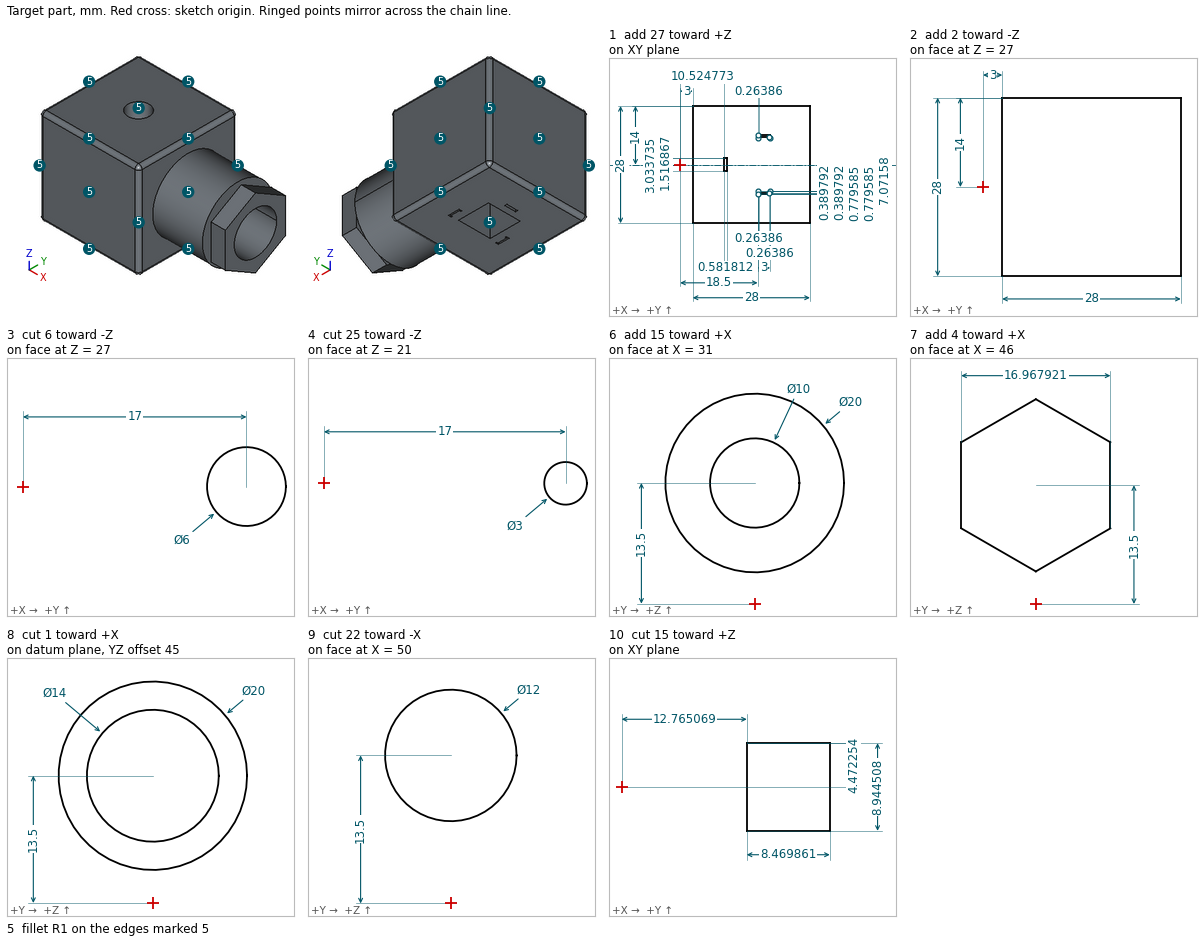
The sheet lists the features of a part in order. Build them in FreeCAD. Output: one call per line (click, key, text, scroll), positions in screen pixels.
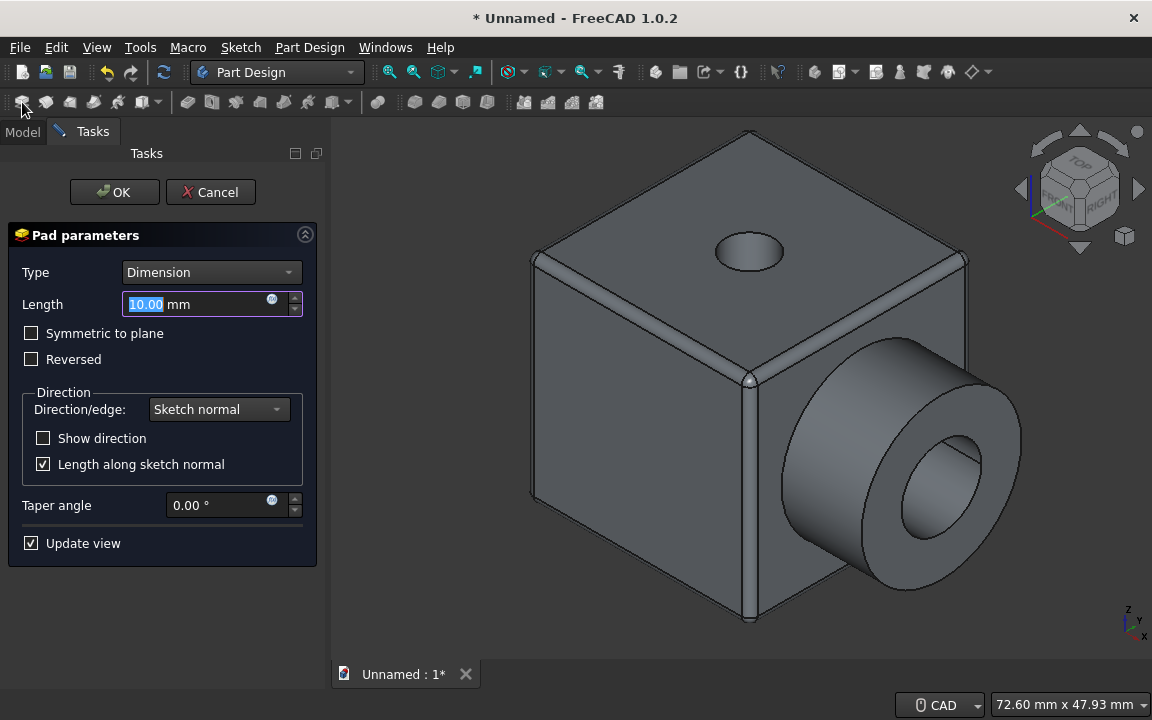
text(15)
key(Tab)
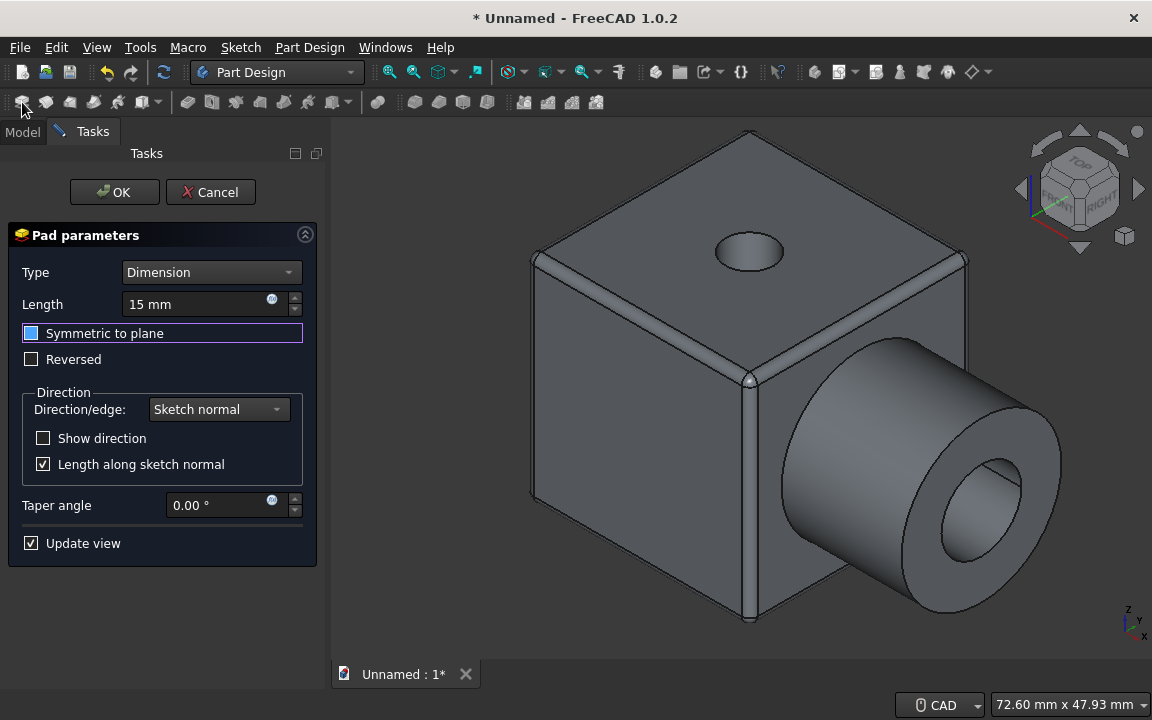
click(115, 192)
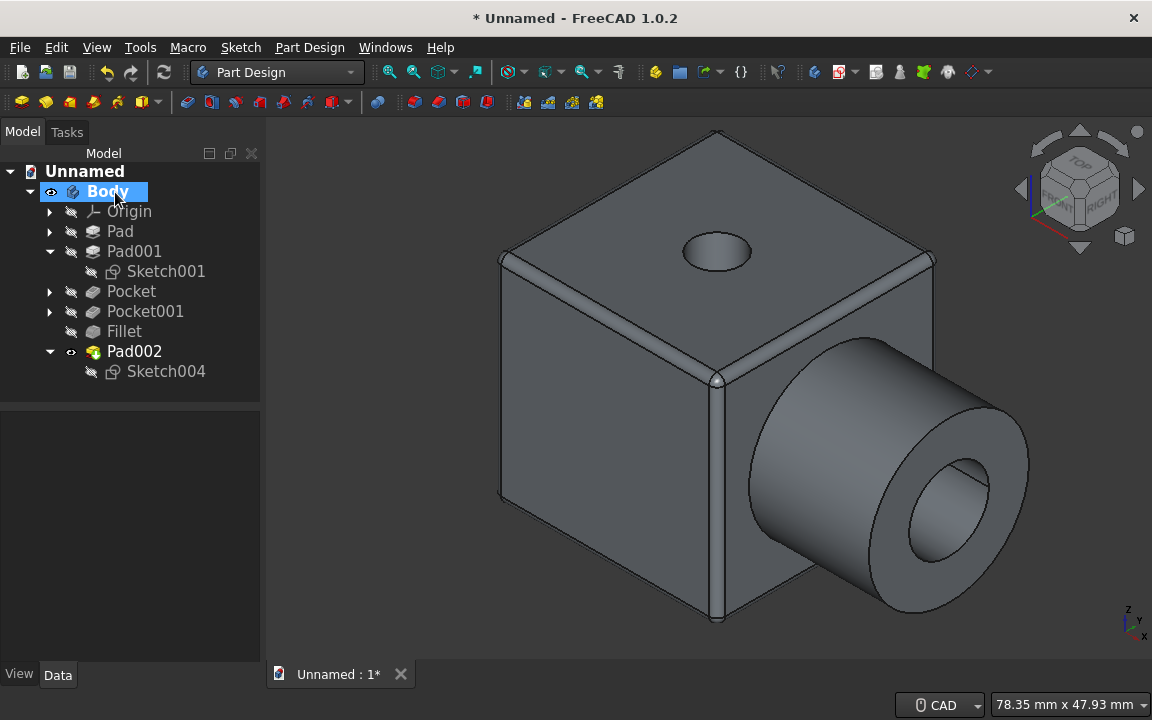
click(390, 72)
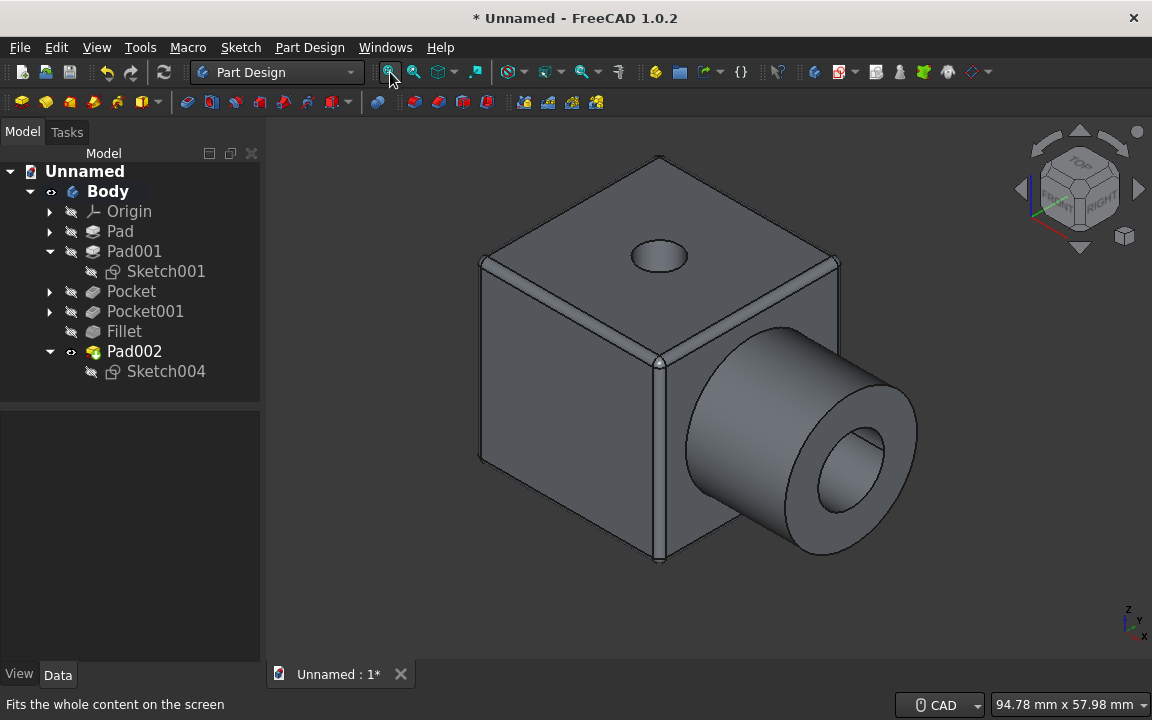
click(813, 534)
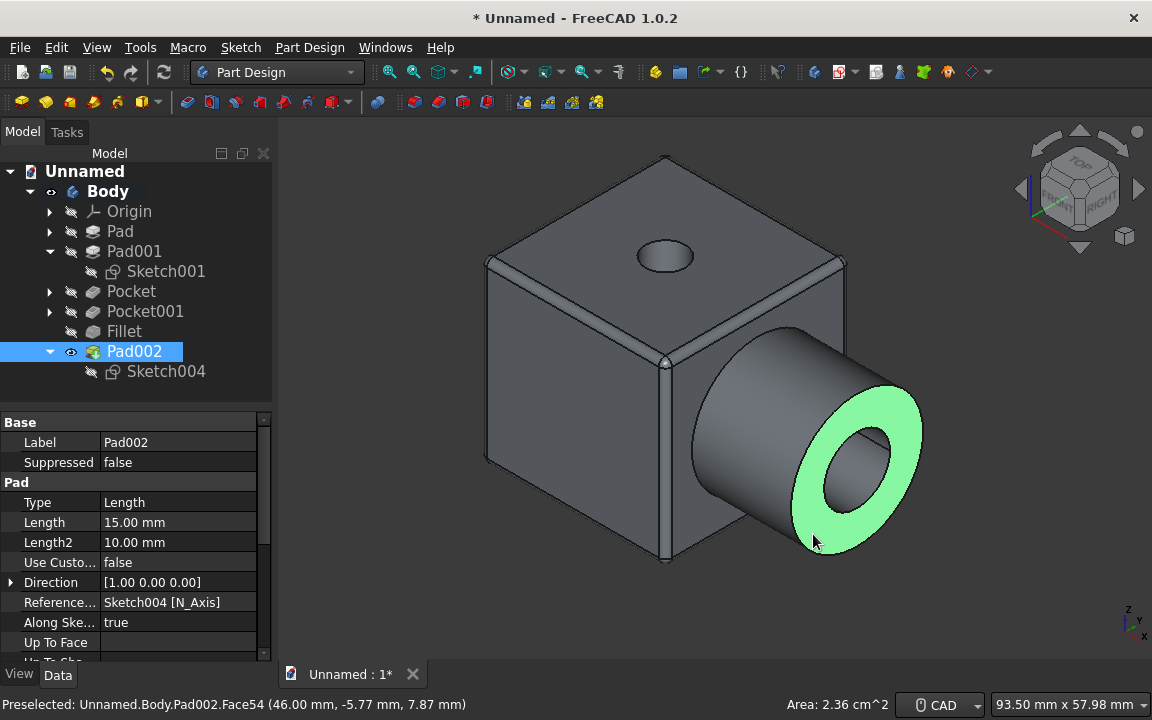
click(840, 72)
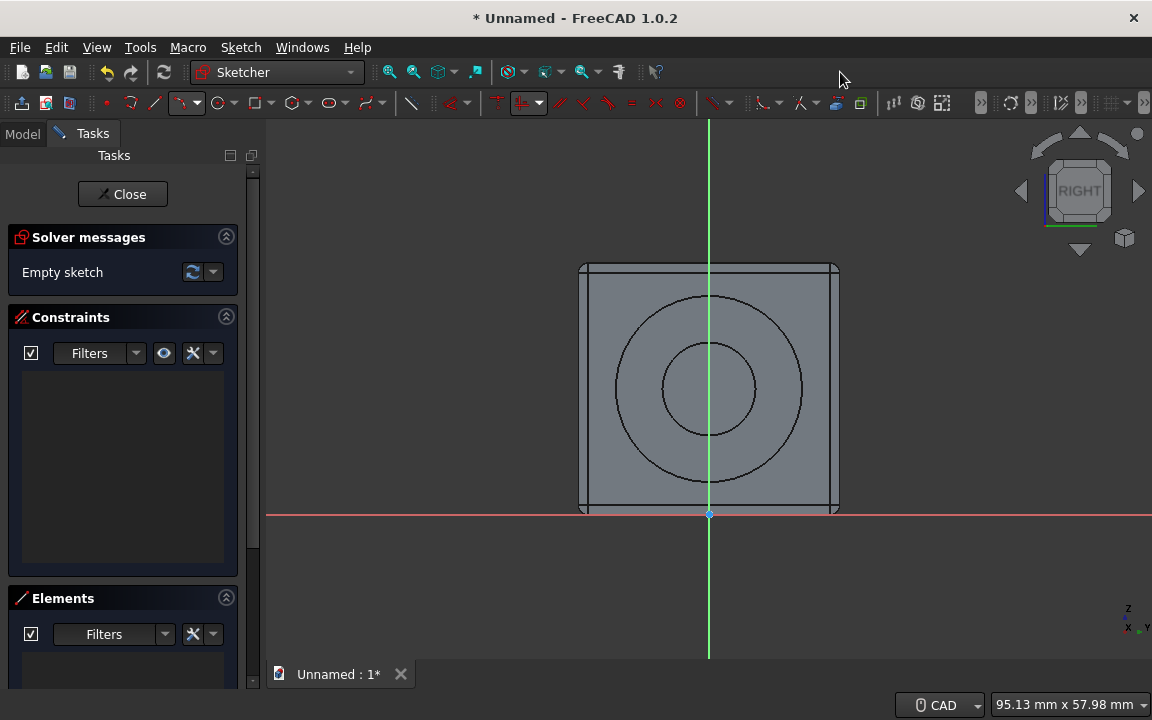
scroll(848, 441, up, 2)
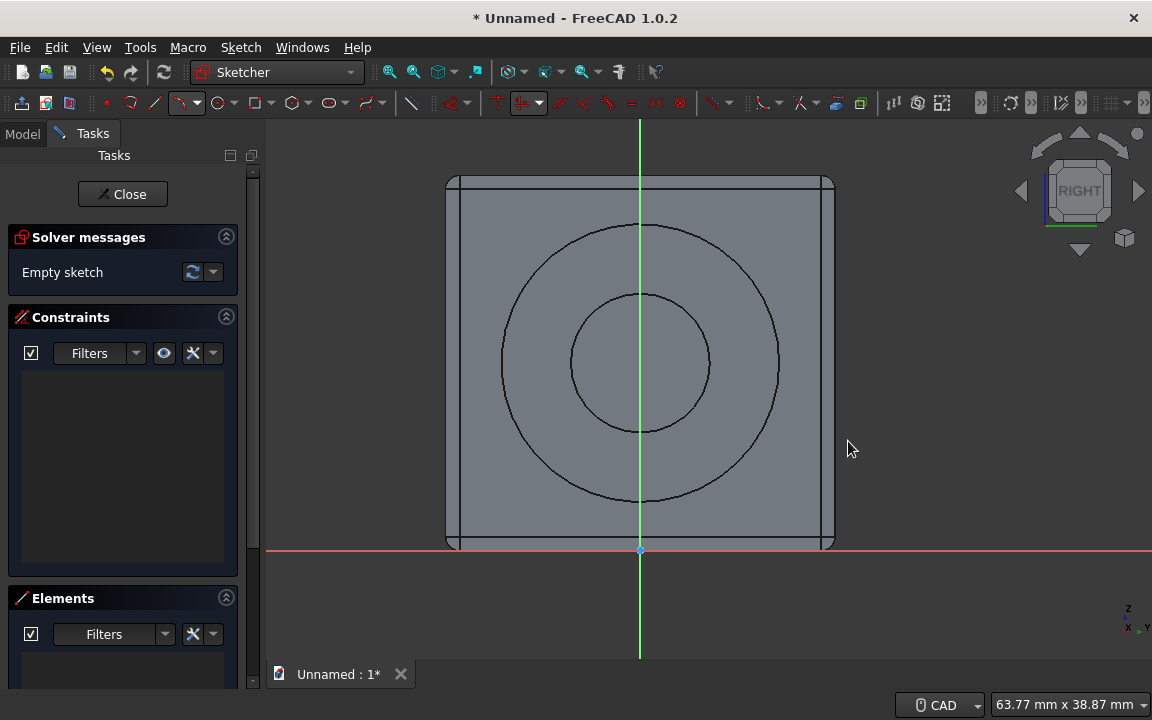
click(292, 104)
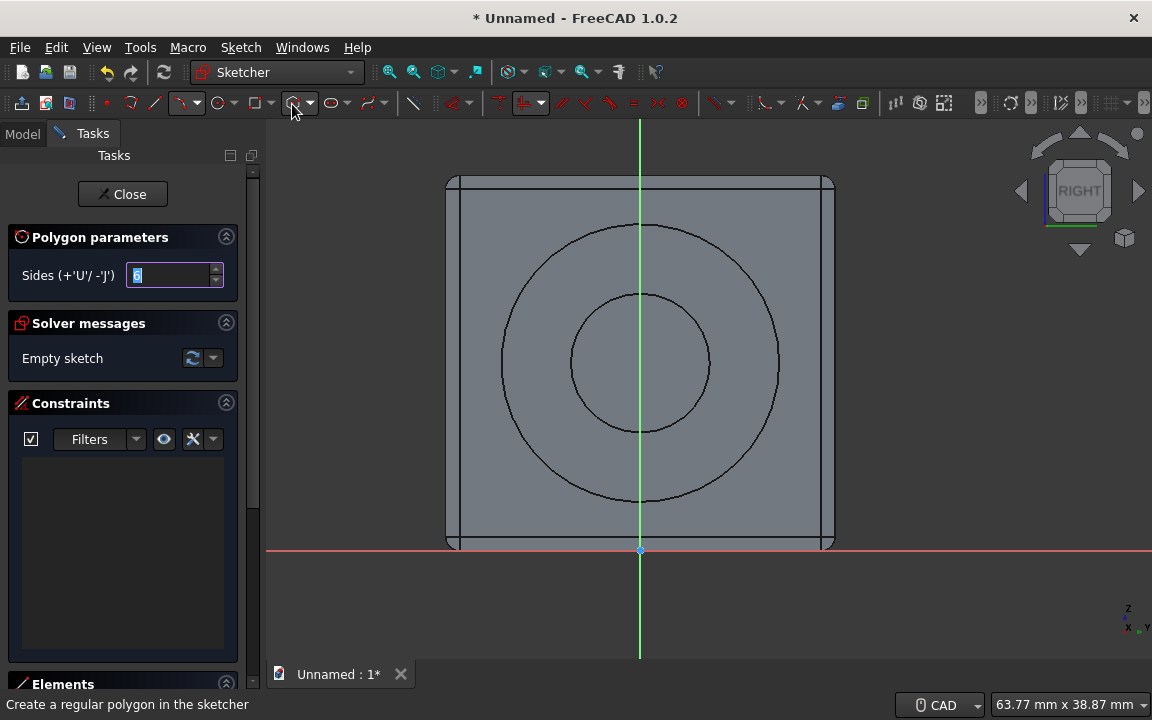
click(640, 363)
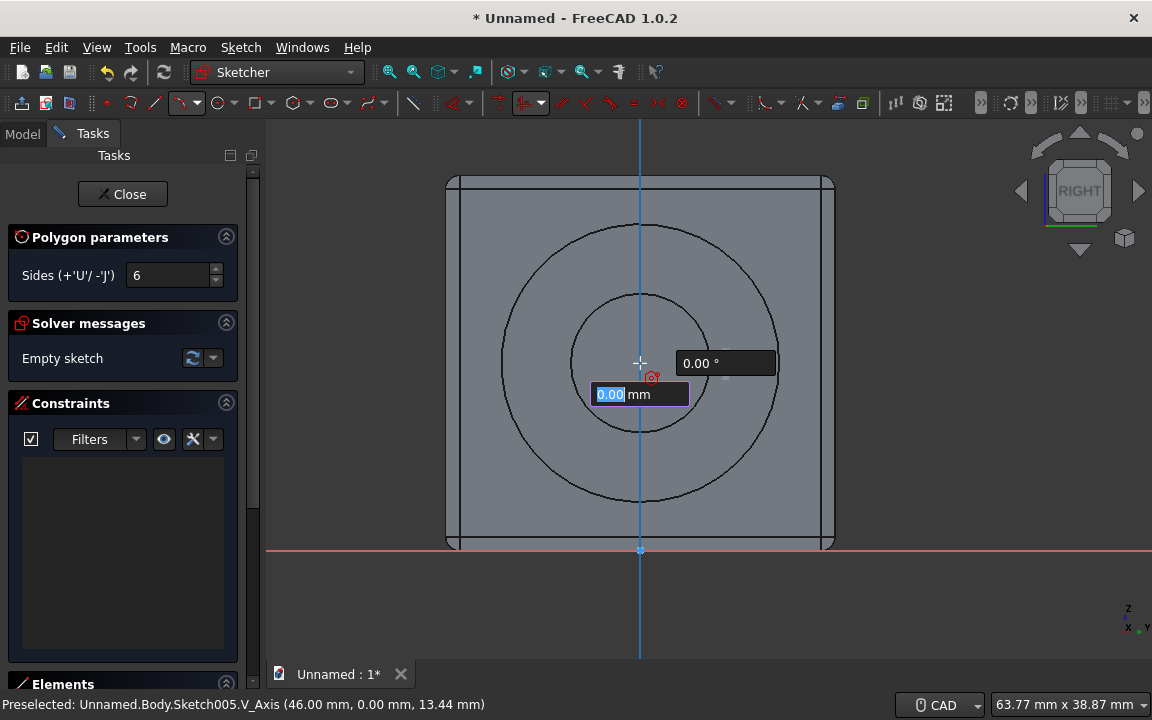
click(640, 227)
right_click(640, 227)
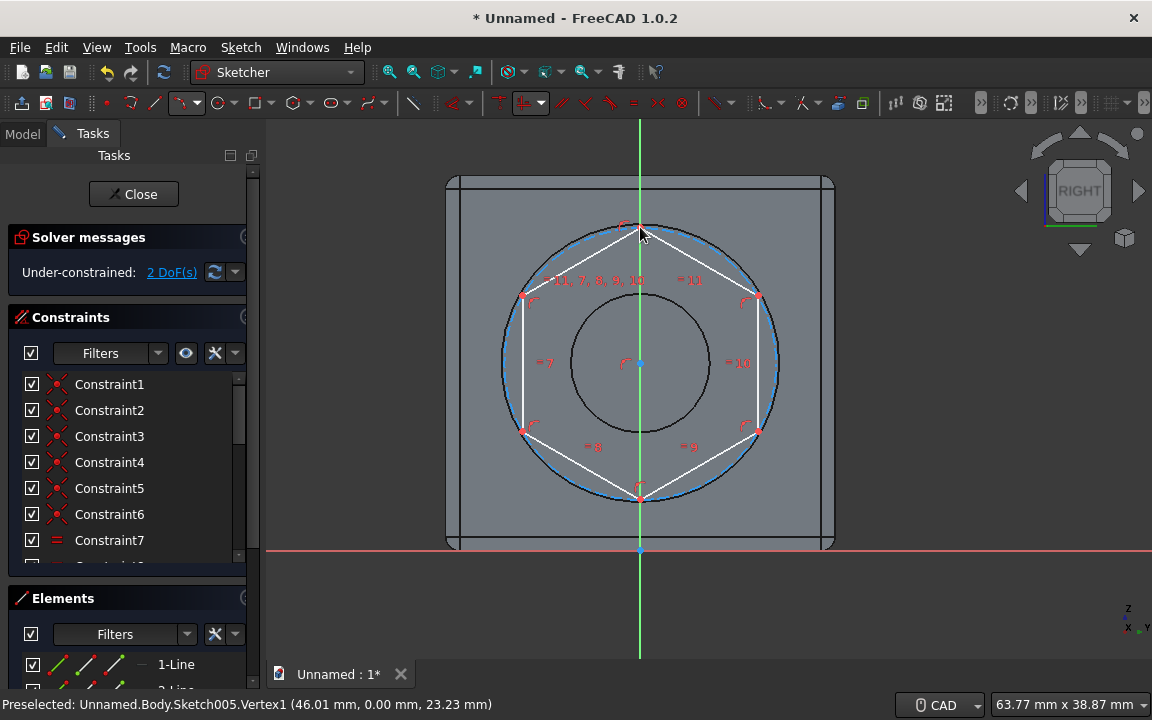
click(452, 104)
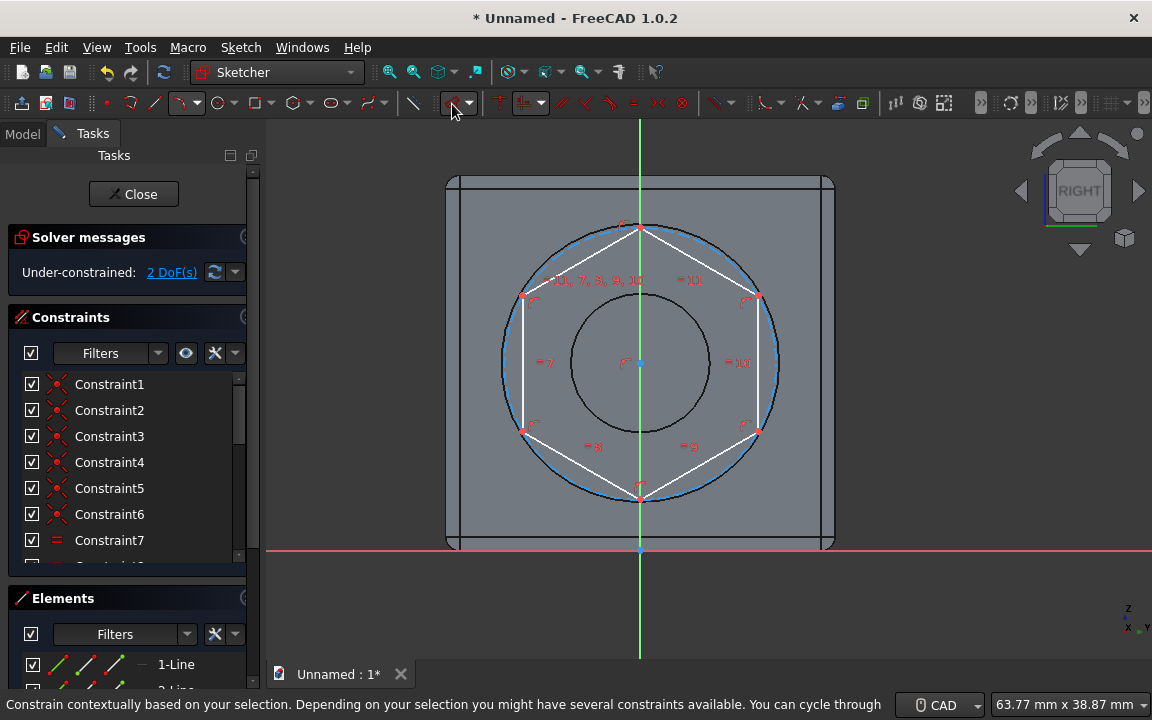
click(640, 364)
click(674, 457)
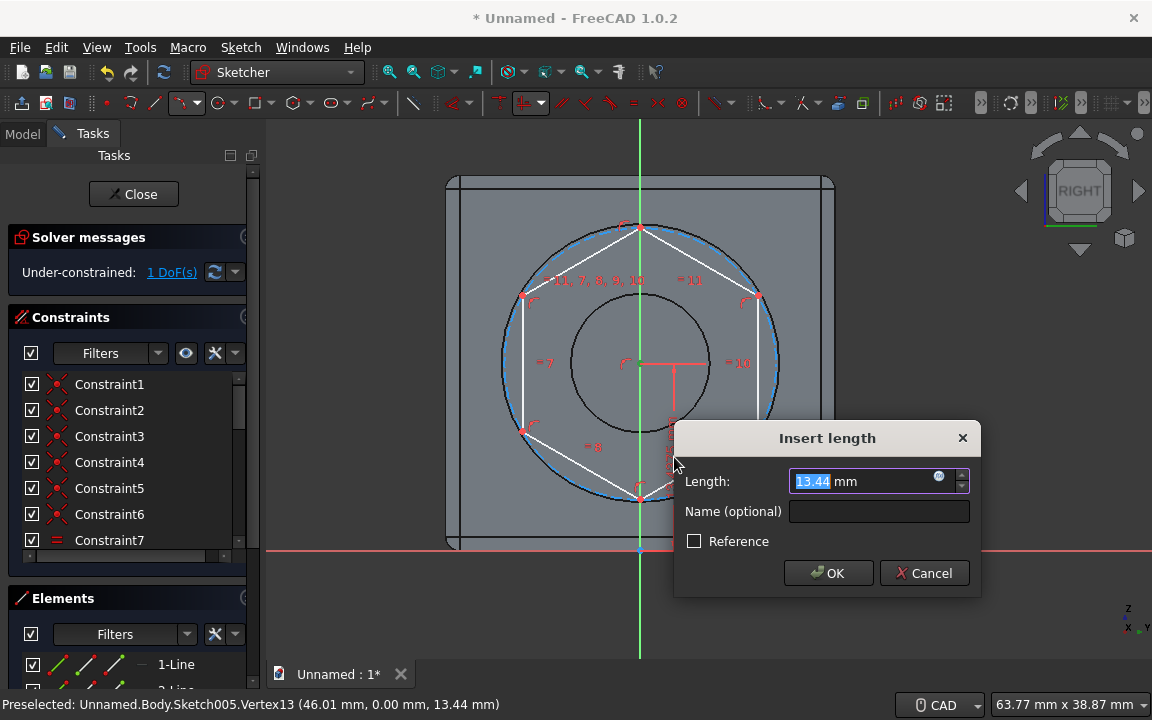
text(13.5)
key(Return)